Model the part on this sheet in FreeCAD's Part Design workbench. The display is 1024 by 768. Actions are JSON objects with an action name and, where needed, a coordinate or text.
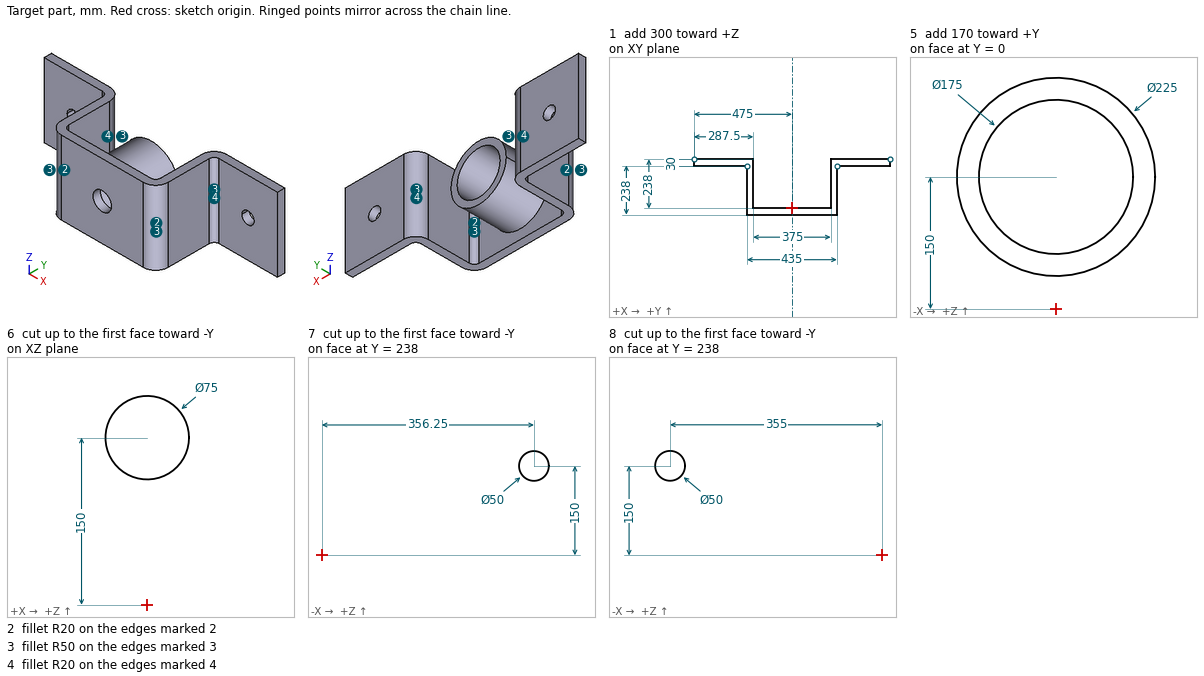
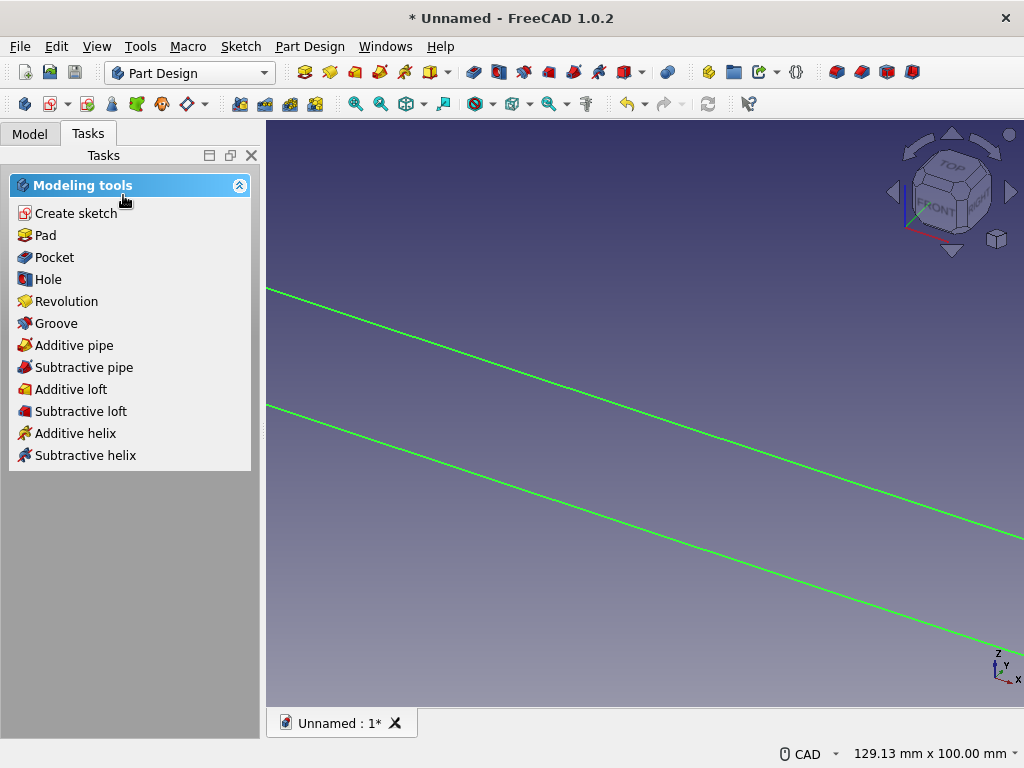
{"action": "left_click", "coordinate": [305, 72]}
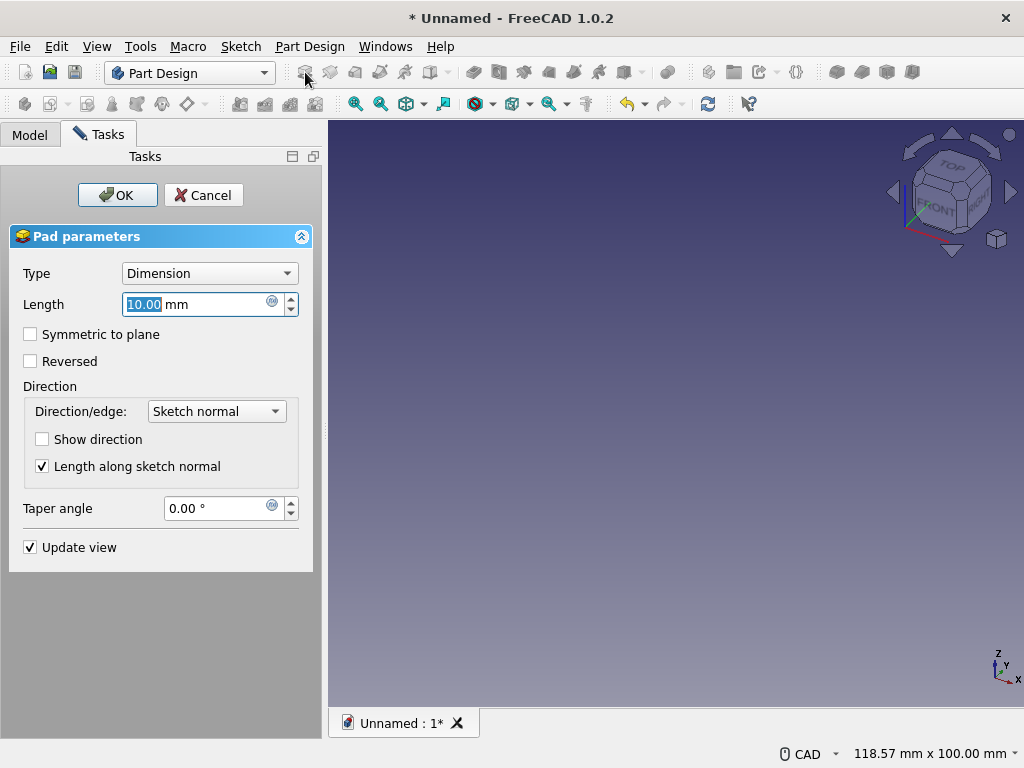
{"action": "type", "text": "300"}
{"action": "key", "text": "Tab"}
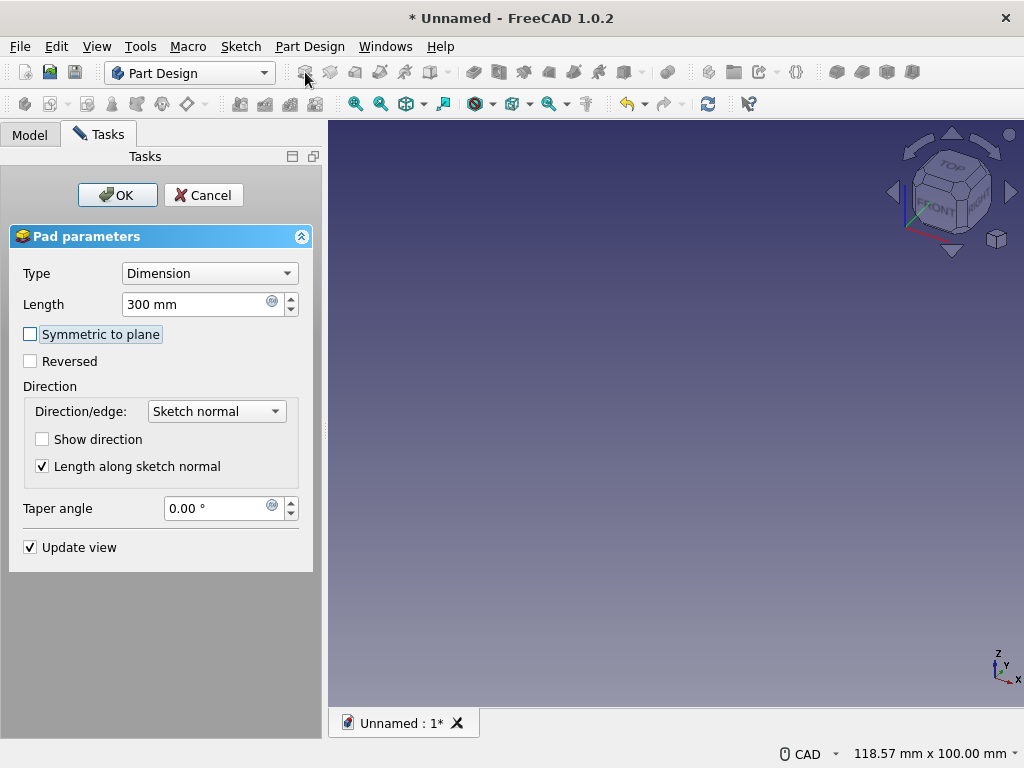
{"action": "left_click", "coordinate": [118, 195]}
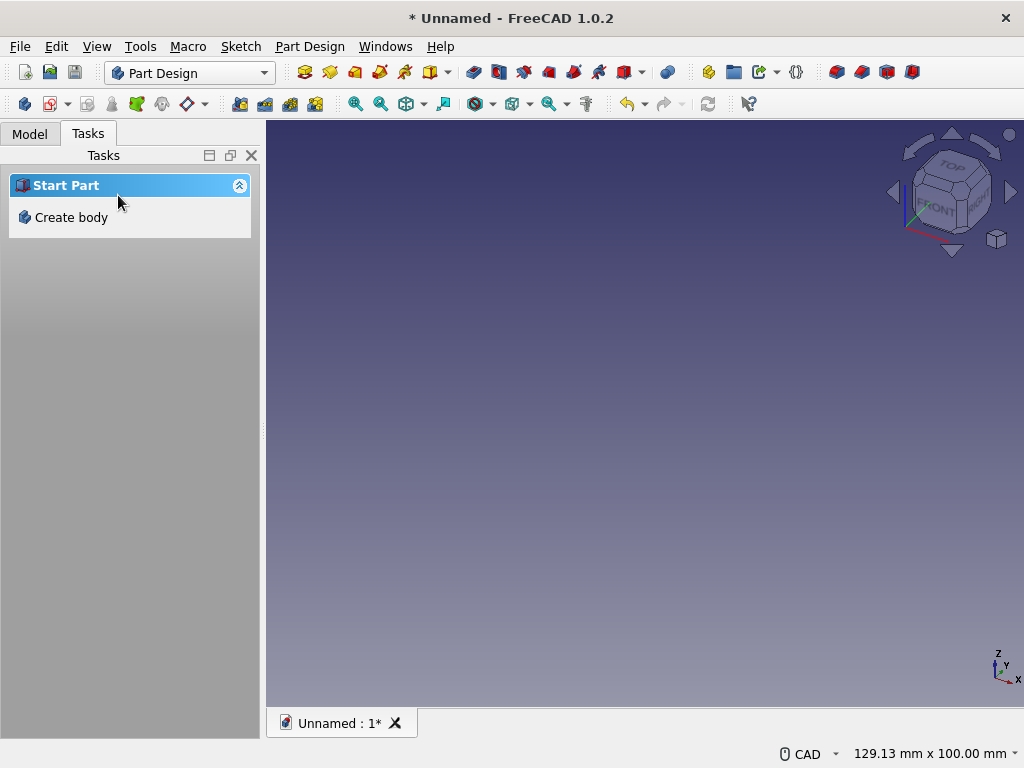
{"action": "left_click", "coordinate": [356, 104]}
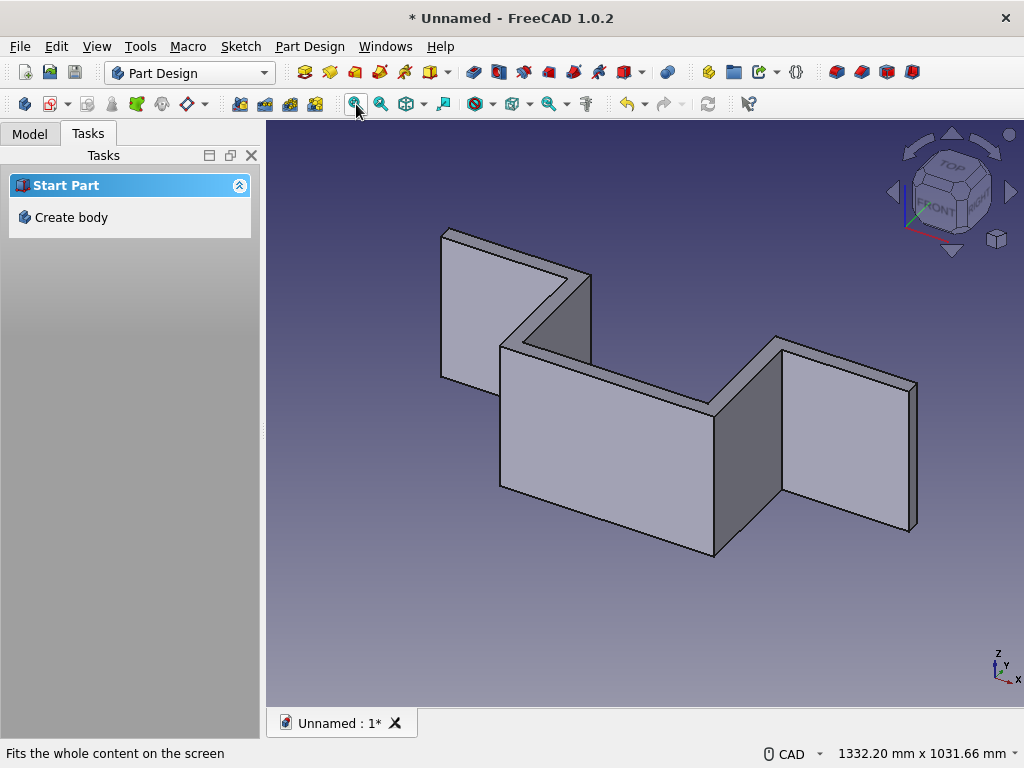
{"action": "key", "text": "0"}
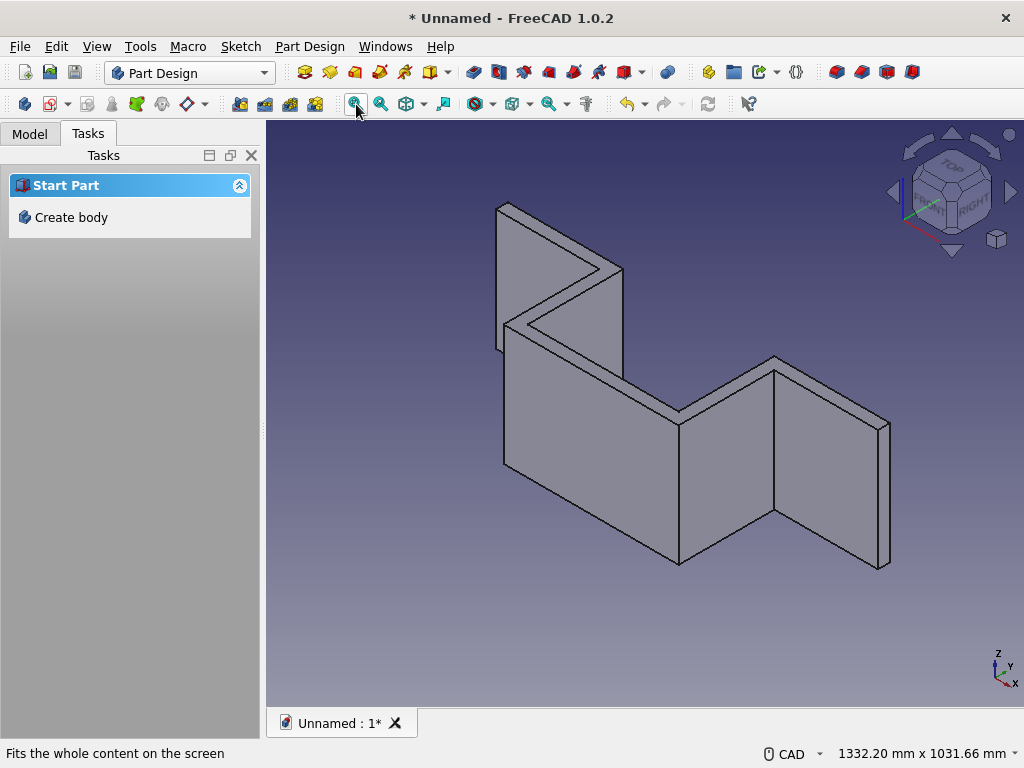
{"action": "key", "text": "2"}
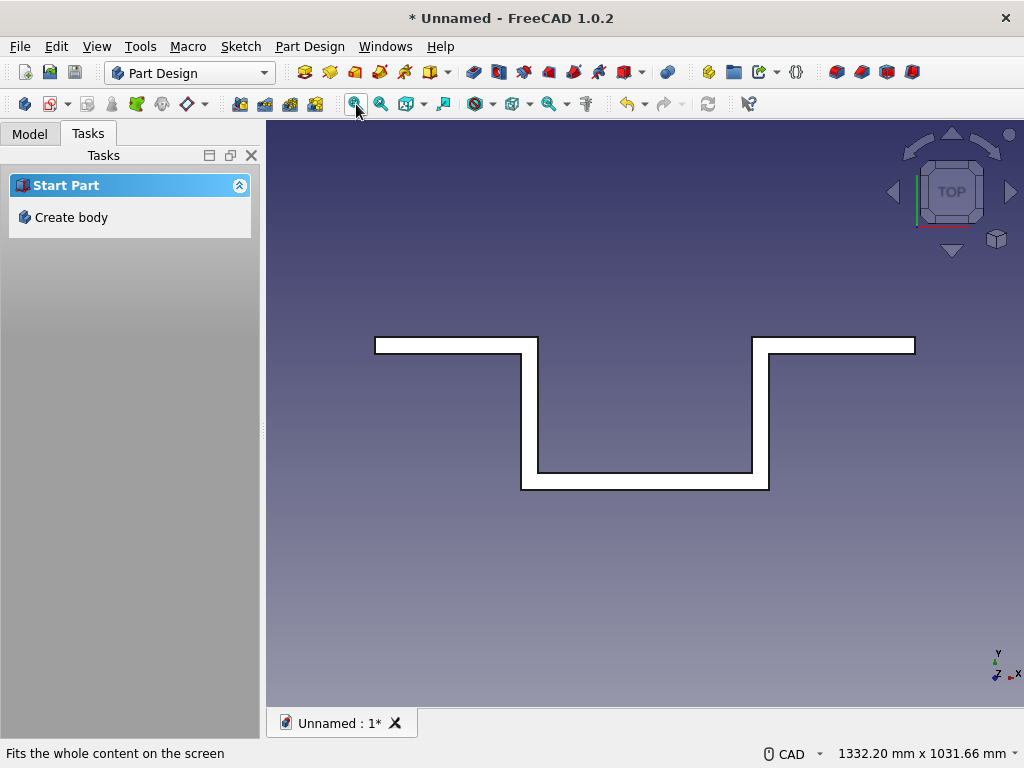
{"action": "key", "text": "1"}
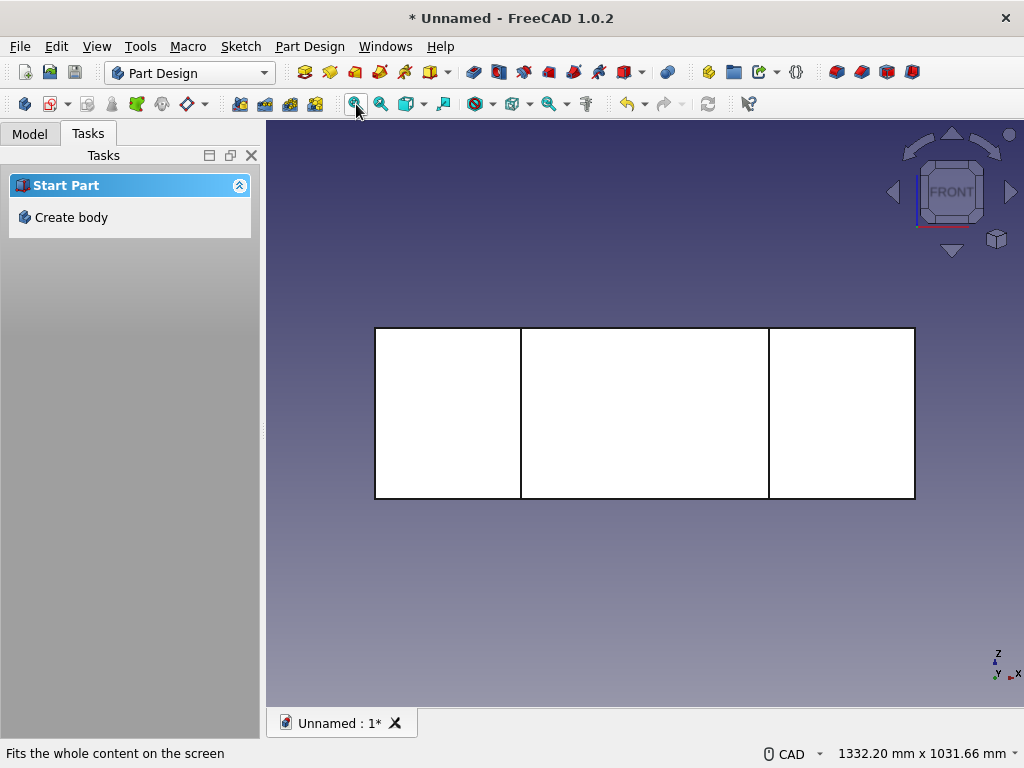
{"action": "key", "text": "3"}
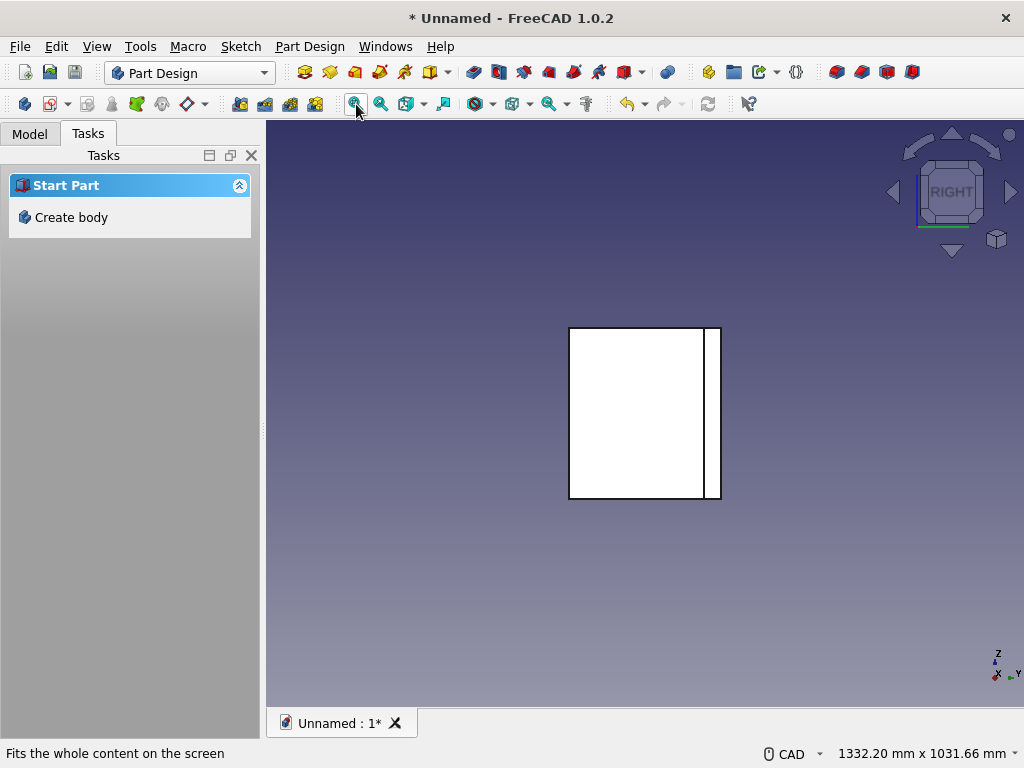
{"action": "left_click", "coordinate": [356, 104]}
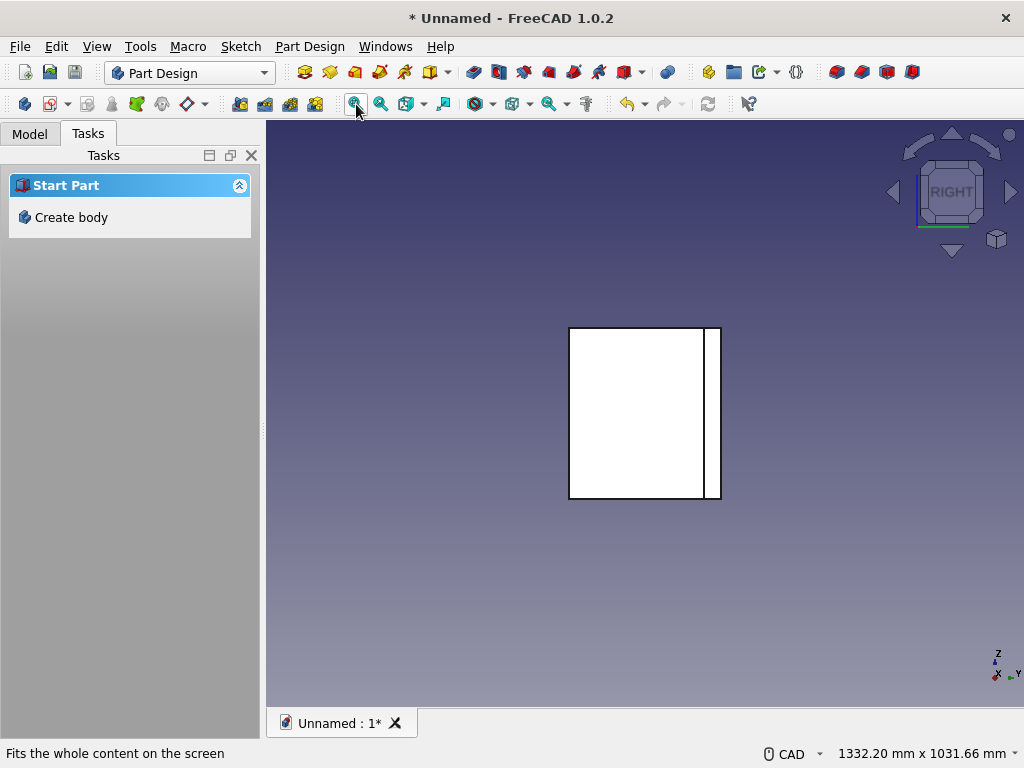
{"action": "key", "text": "5"}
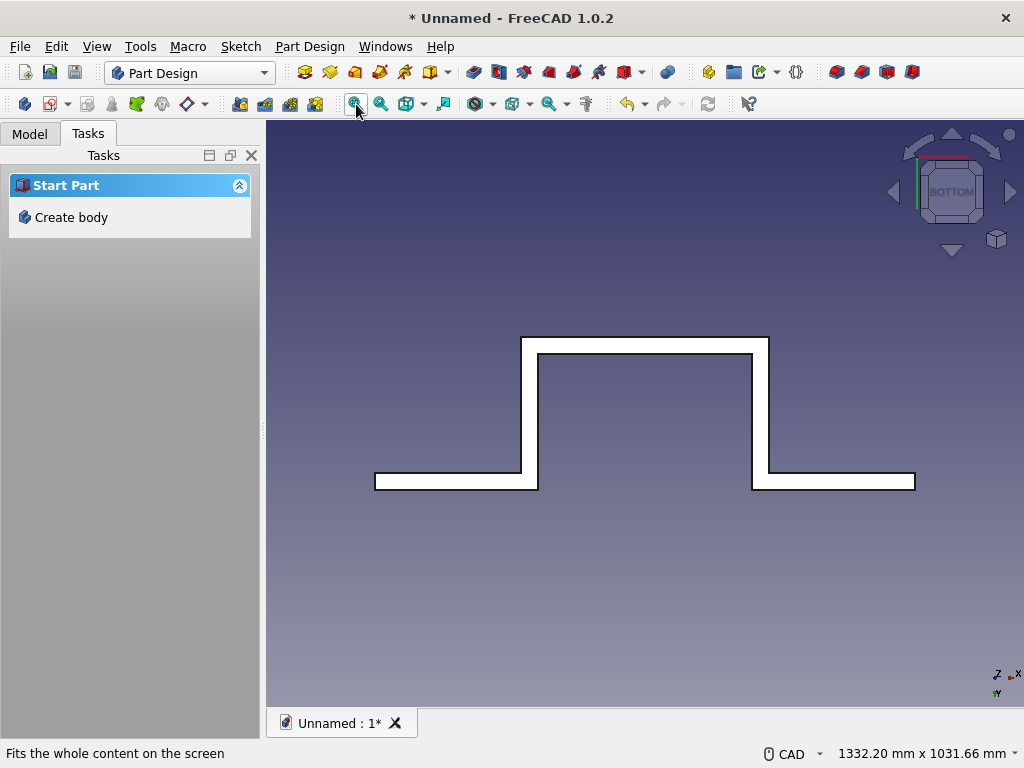
{"action": "key", "text": "4"}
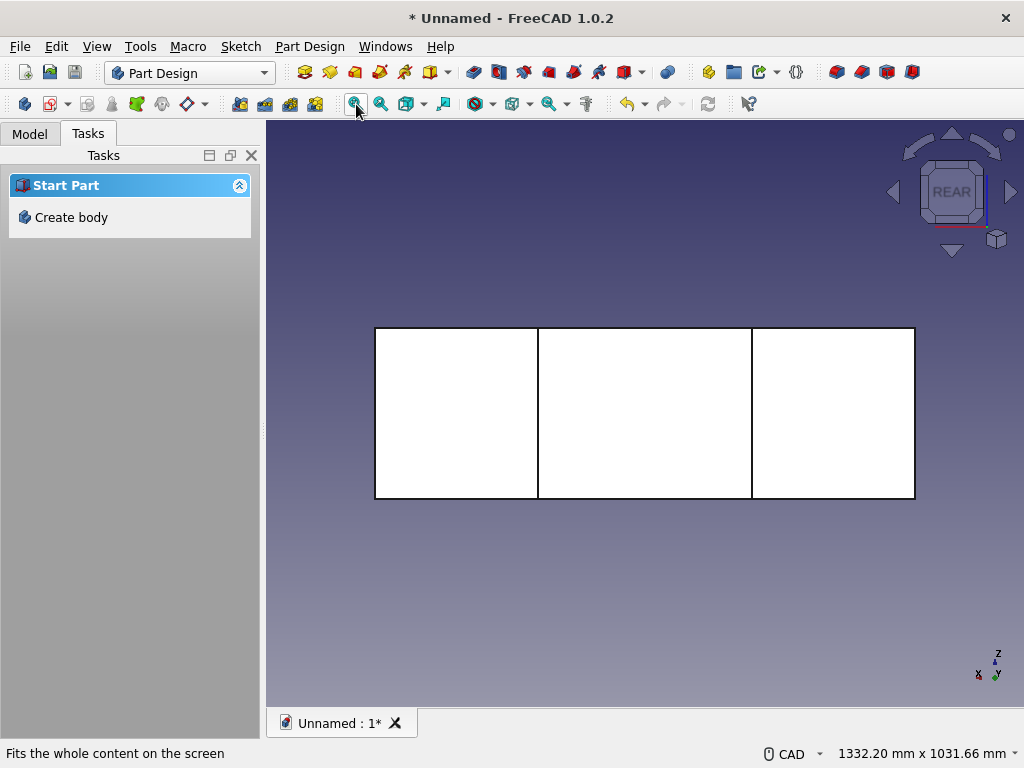
{"action": "key", "text": "6"}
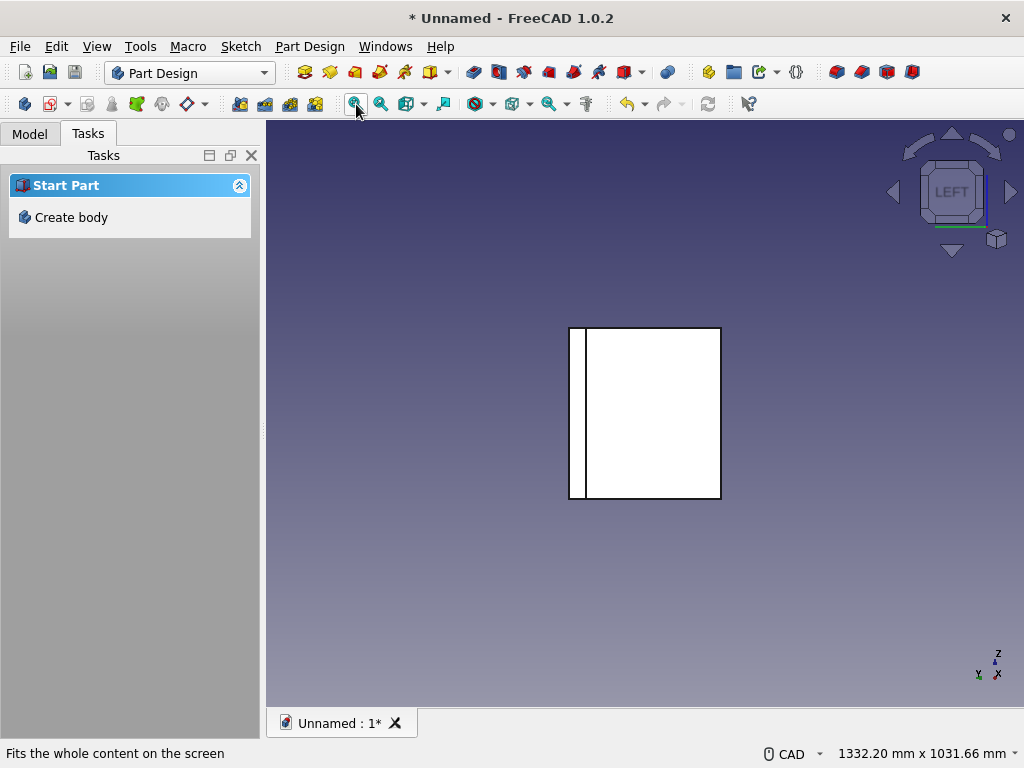
{"action": "left_click", "coordinate": [356, 104]}